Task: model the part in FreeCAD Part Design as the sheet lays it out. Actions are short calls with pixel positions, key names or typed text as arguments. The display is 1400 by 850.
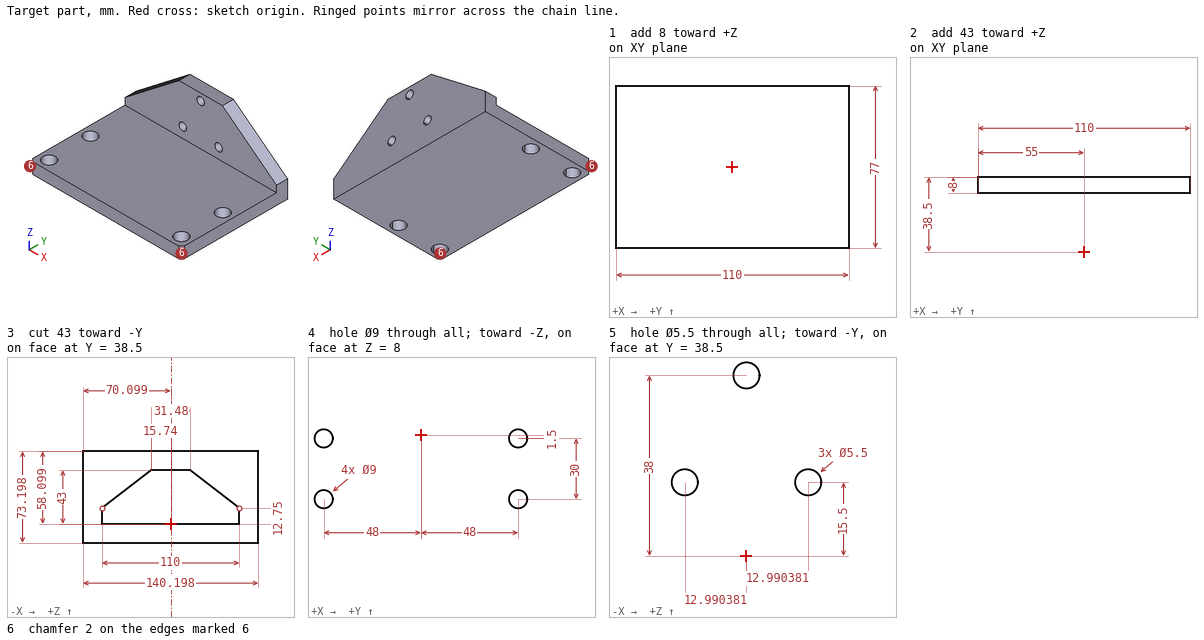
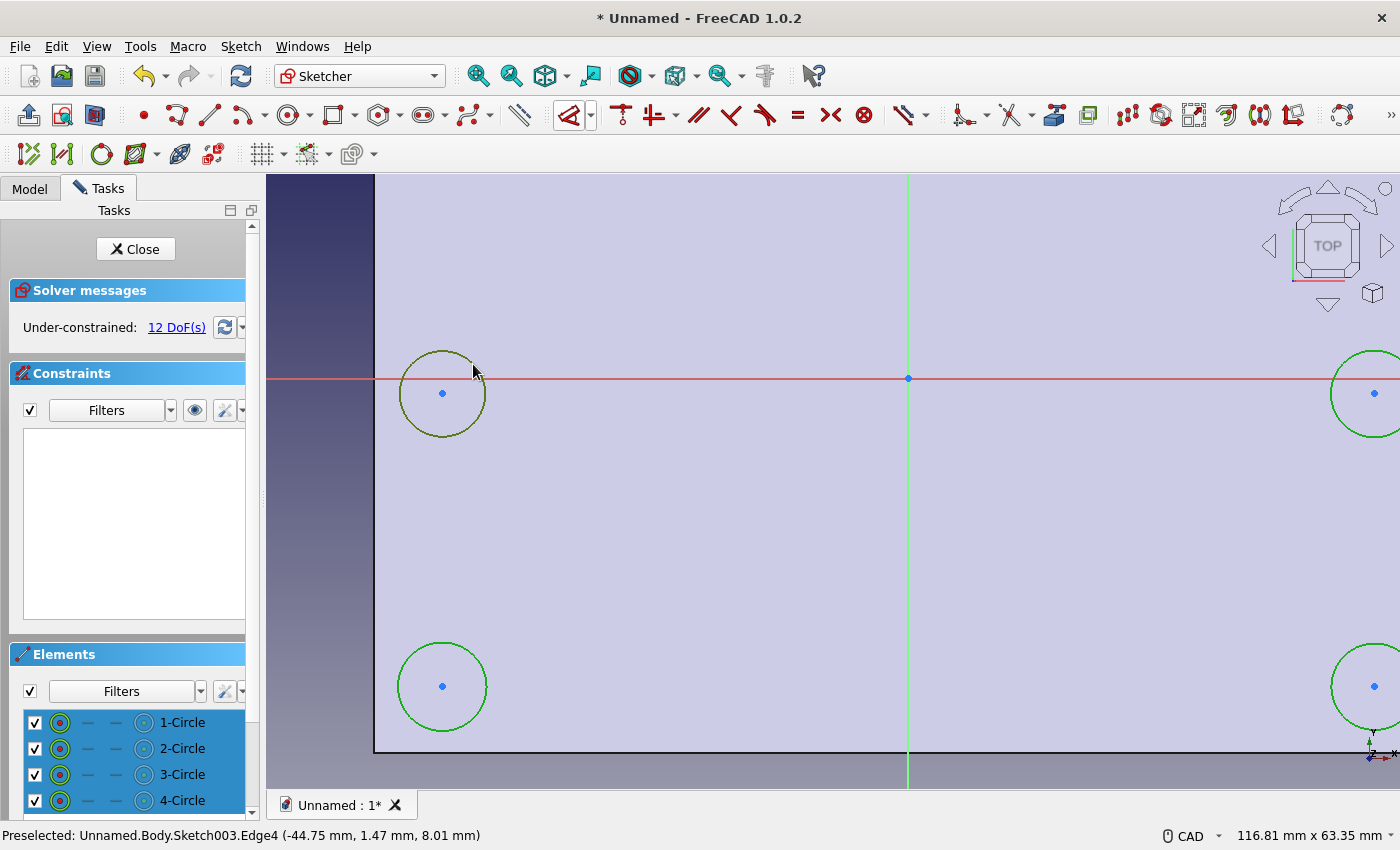
key(e)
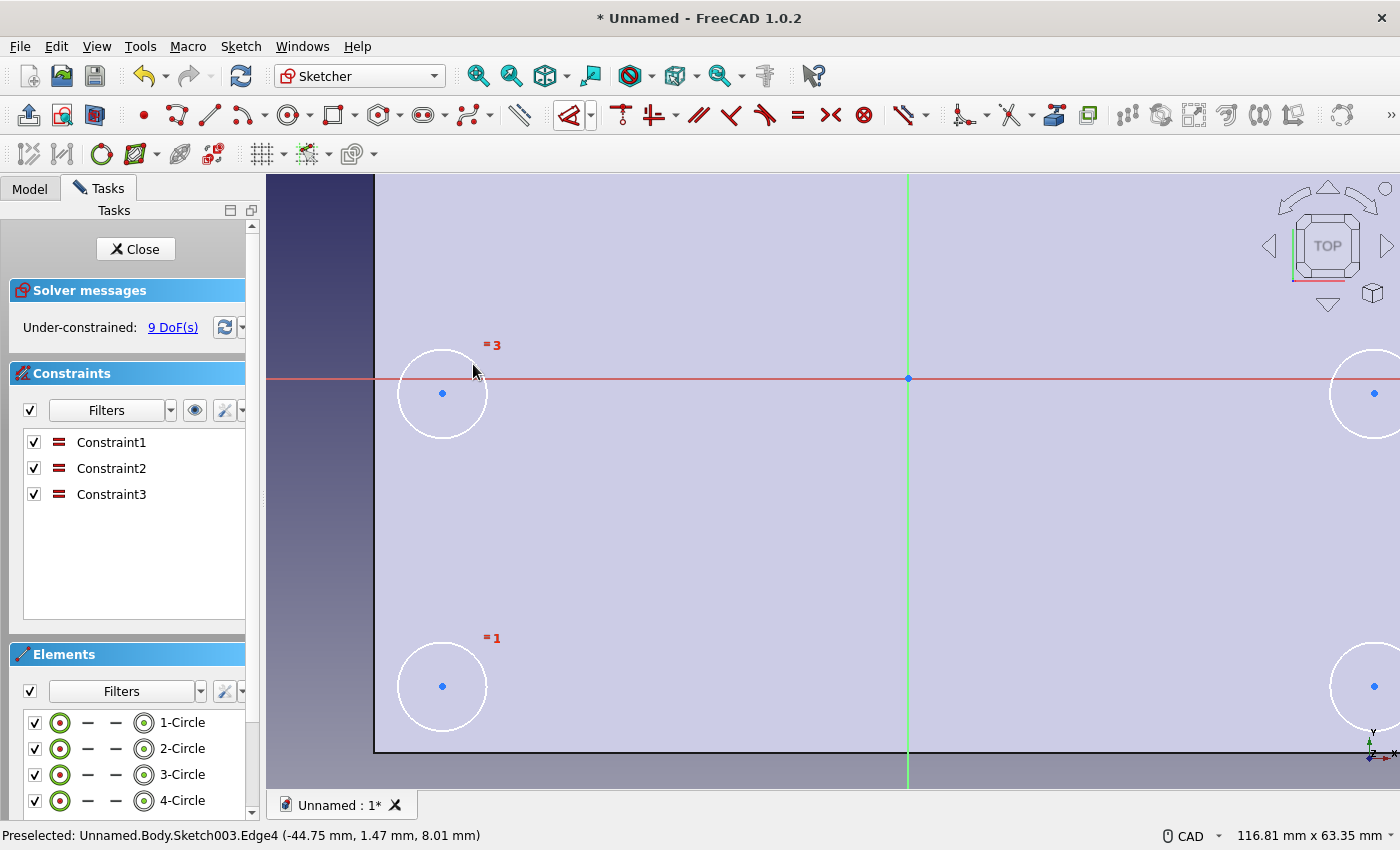
click(442, 687)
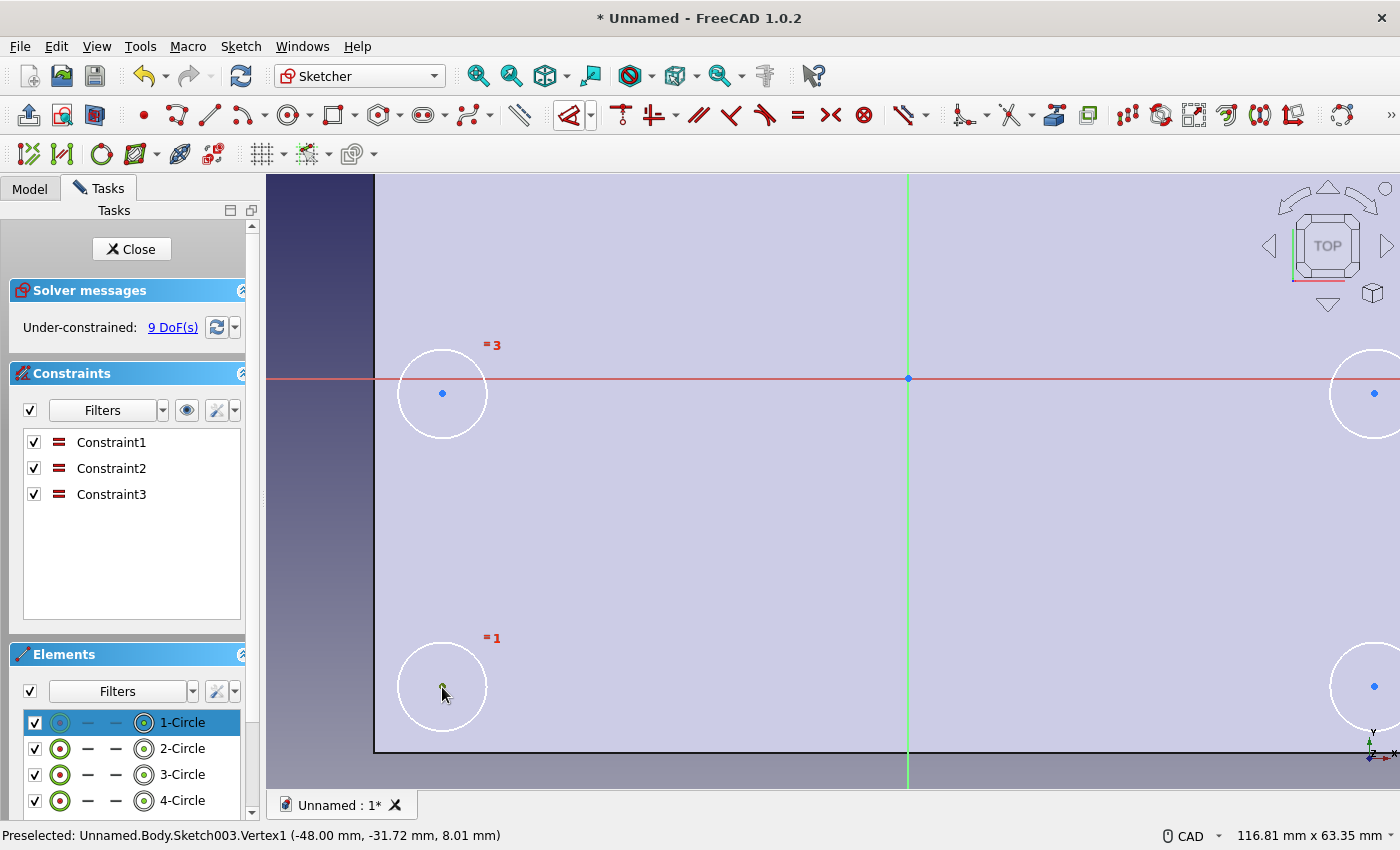
scroll(472, 364, down, 2)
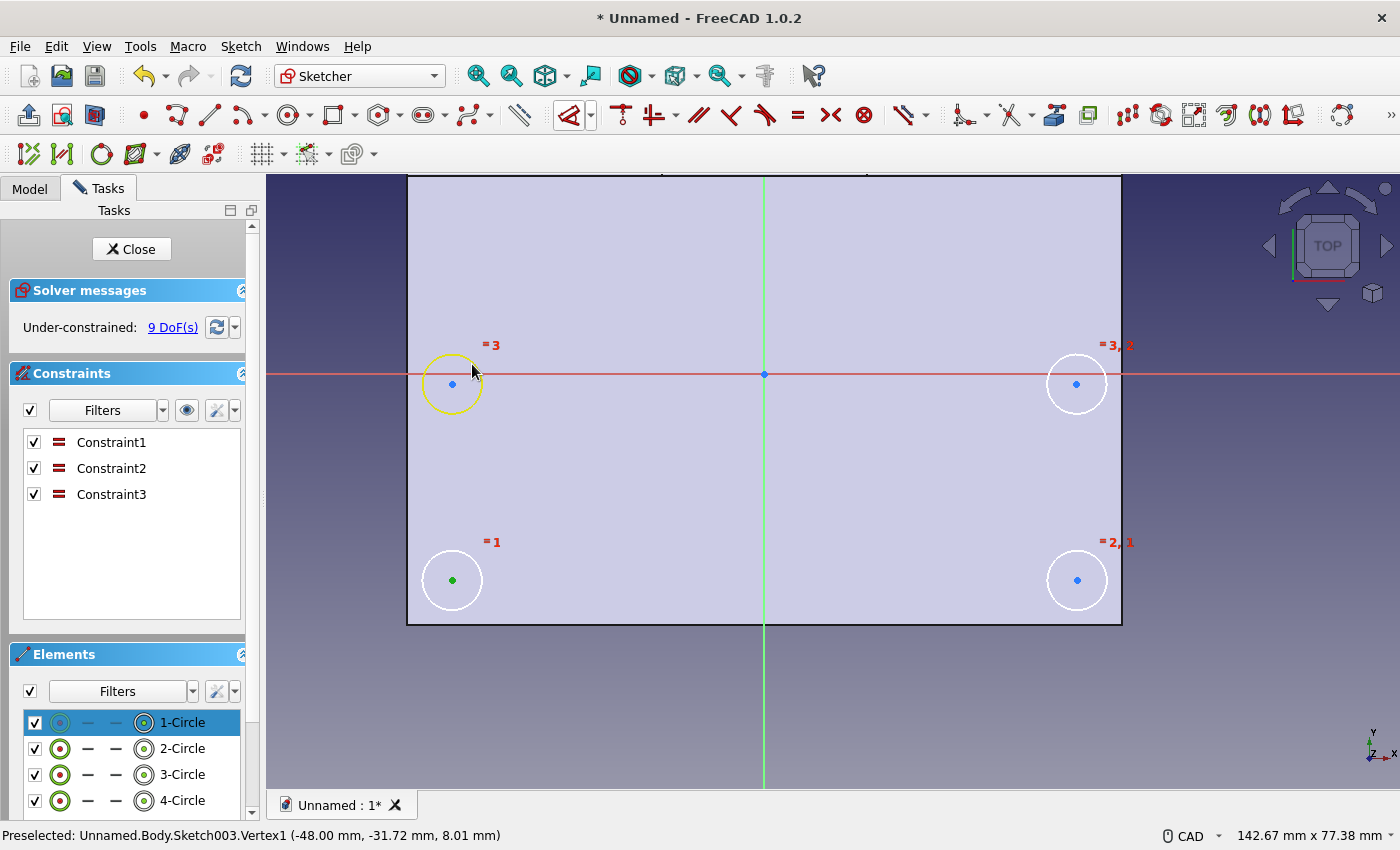
click(1077, 580)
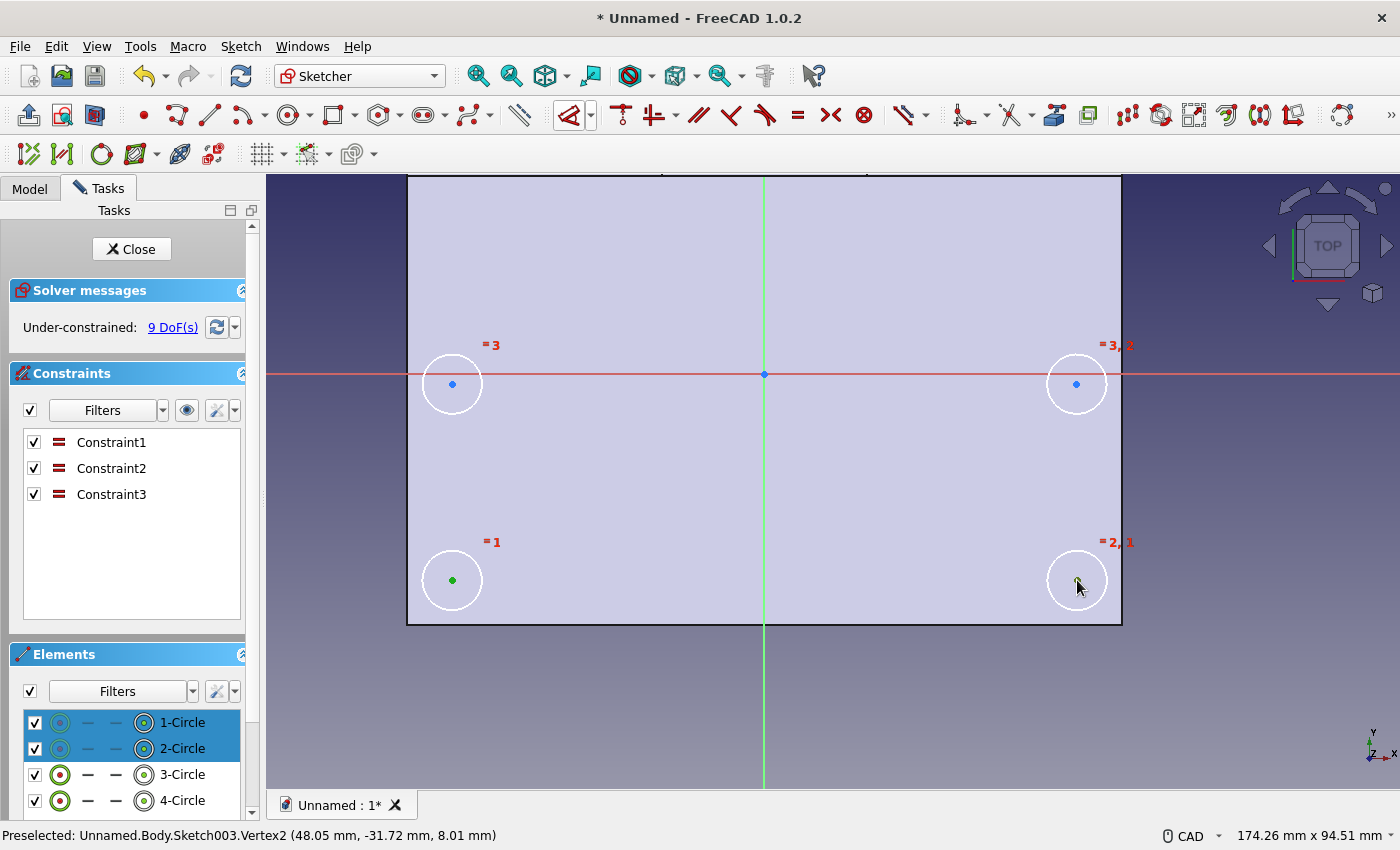
key(h)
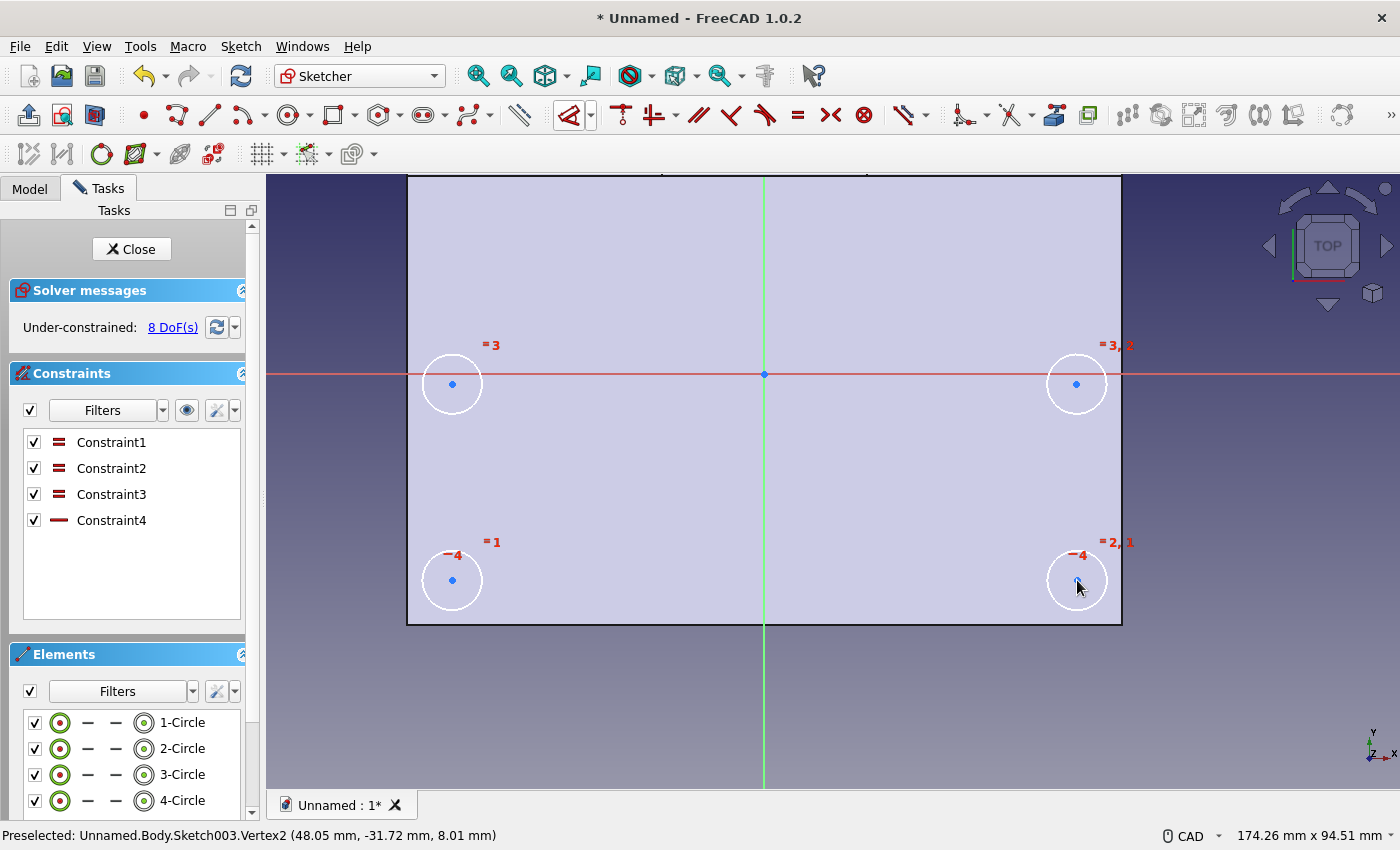
click(1077, 580)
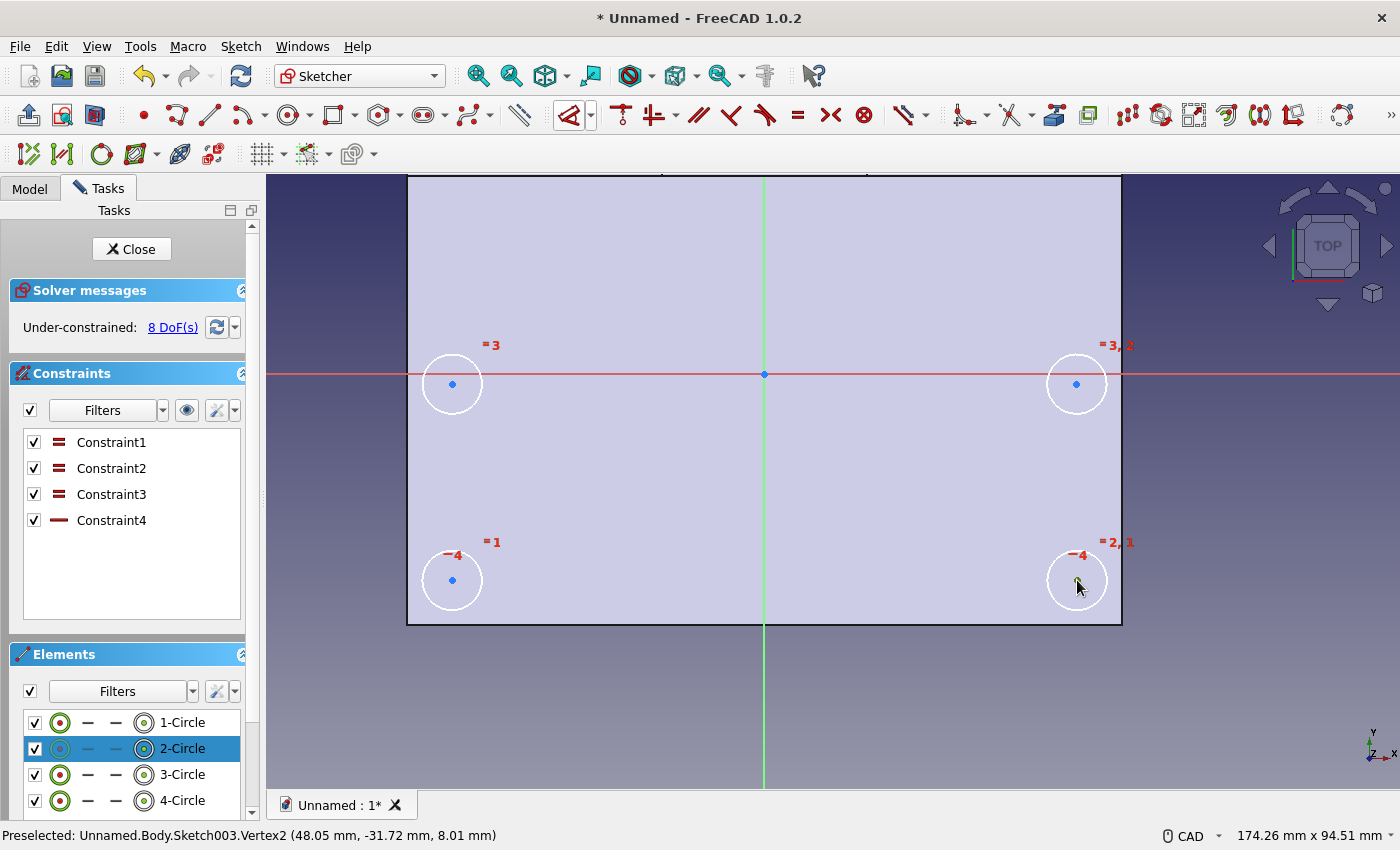
click(1077, 384)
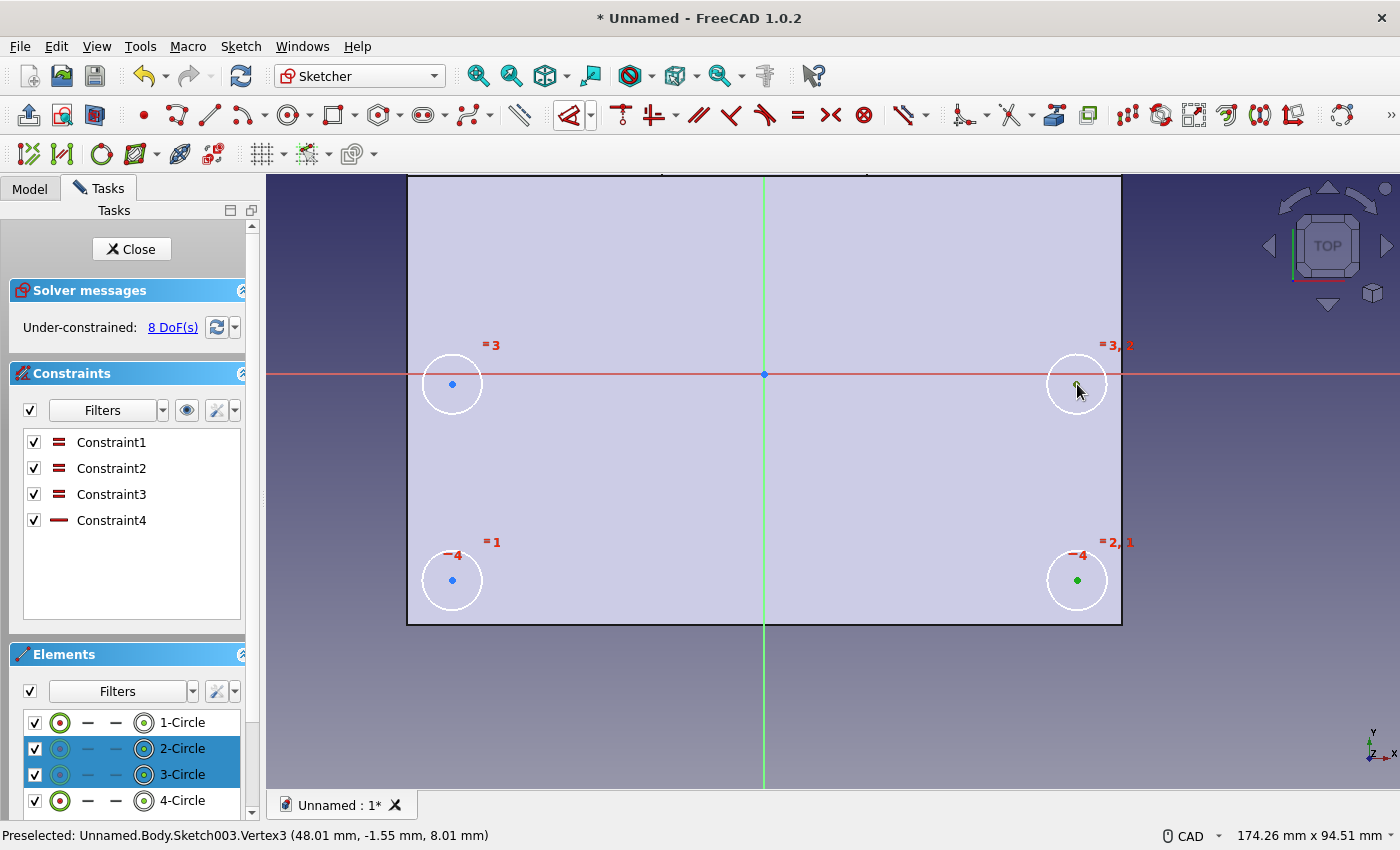
key(v)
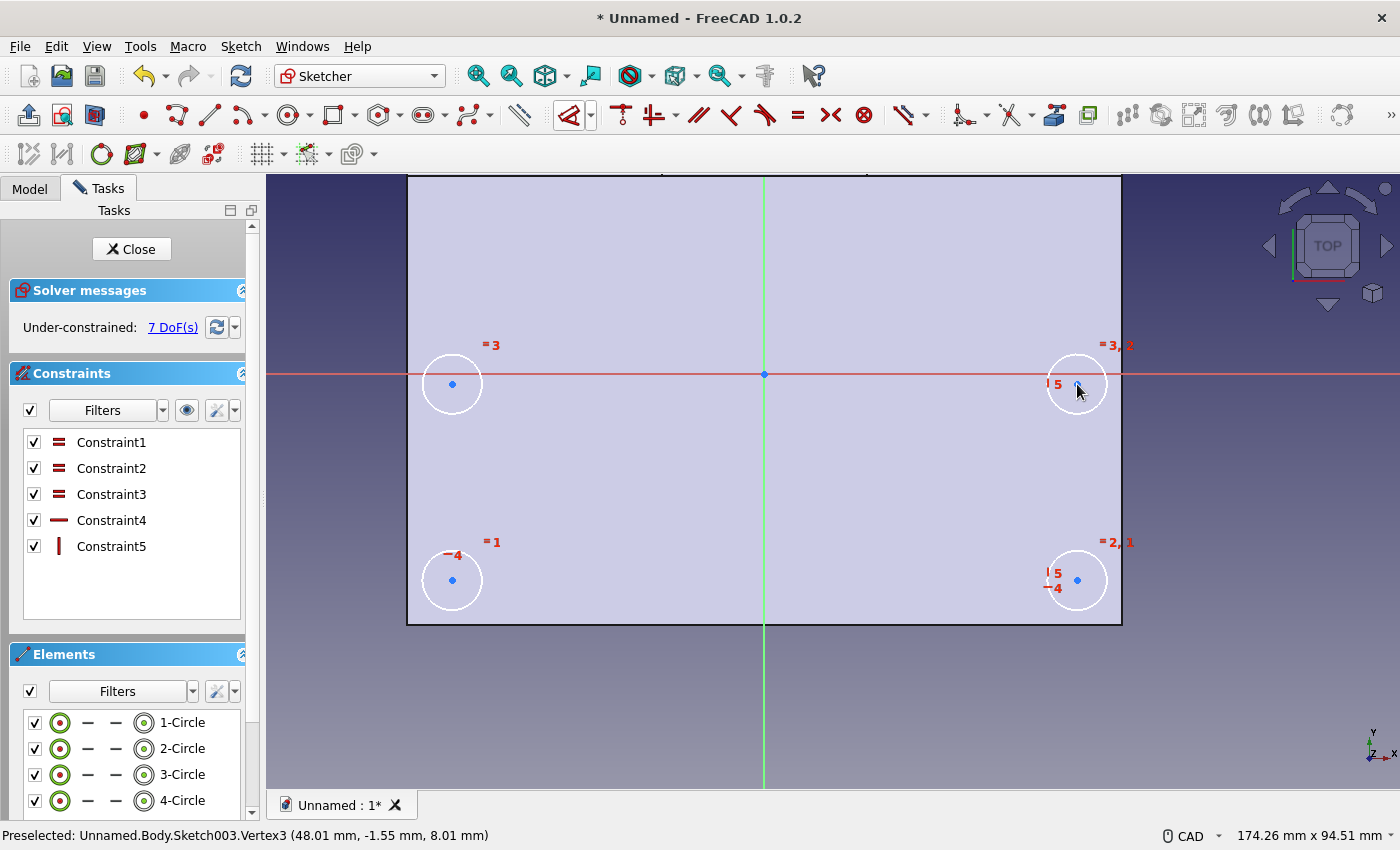
click(452, 580)